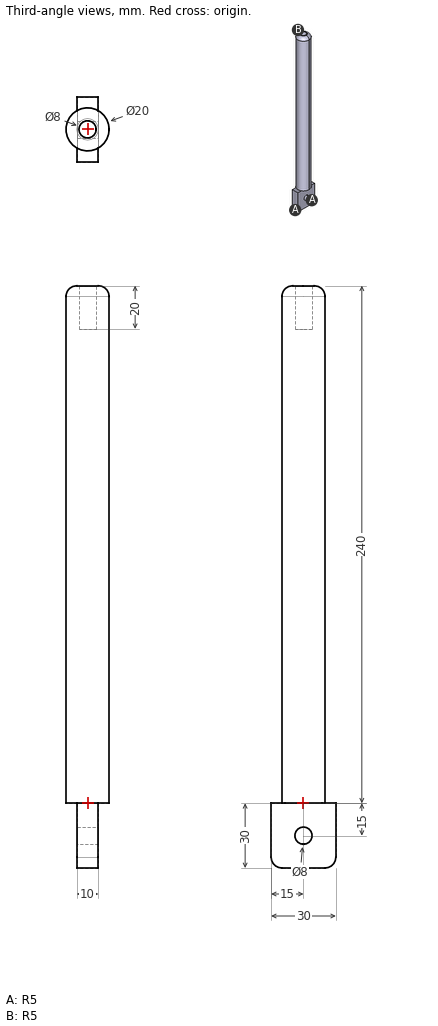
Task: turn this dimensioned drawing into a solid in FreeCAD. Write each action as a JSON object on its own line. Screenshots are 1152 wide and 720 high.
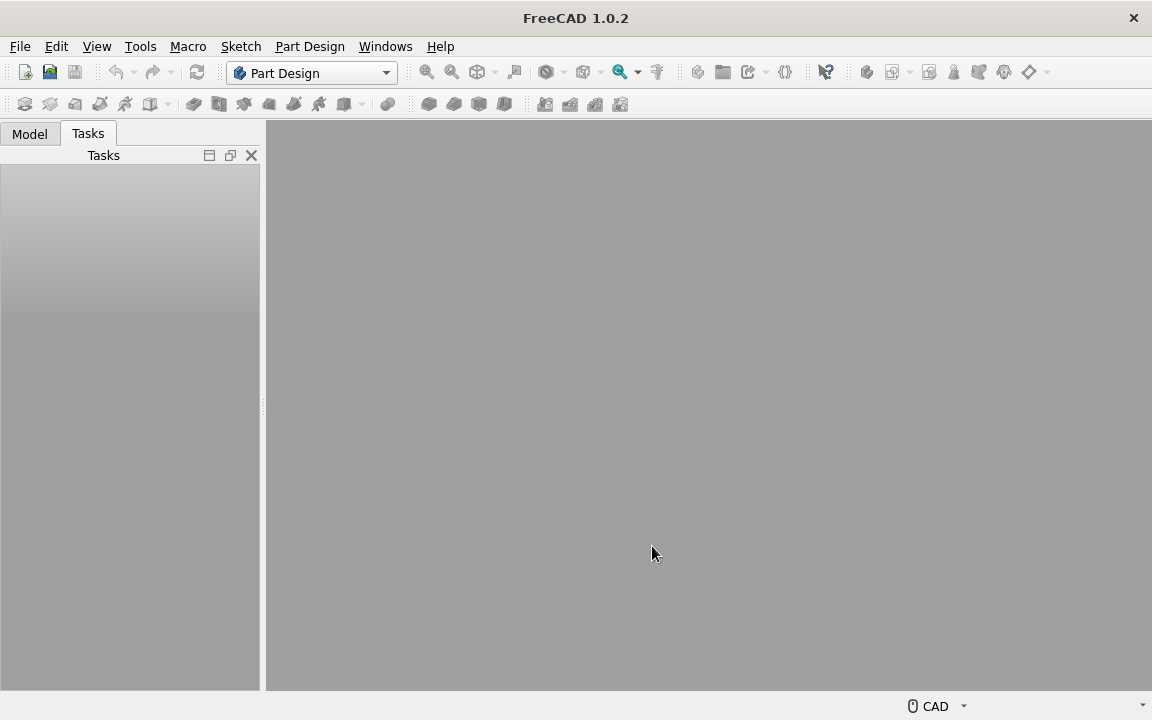
{"action": "key", "text": "ctrl+n"}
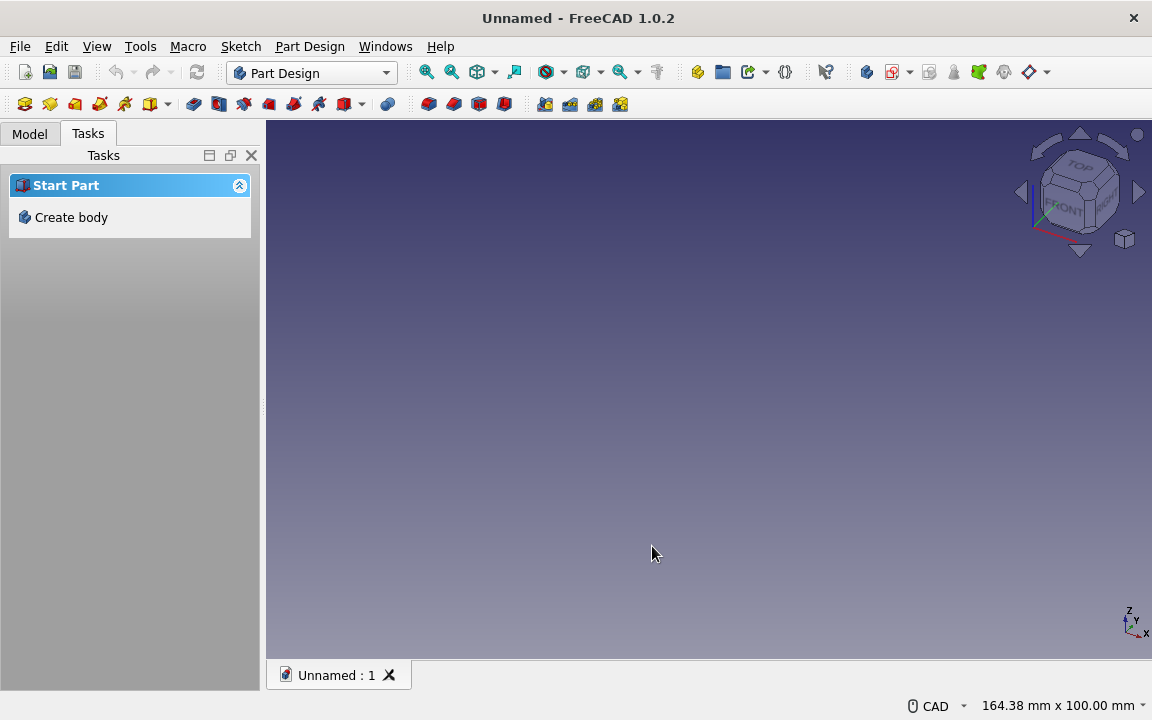
{"action": "left_click", "coordinate": [892, 72]}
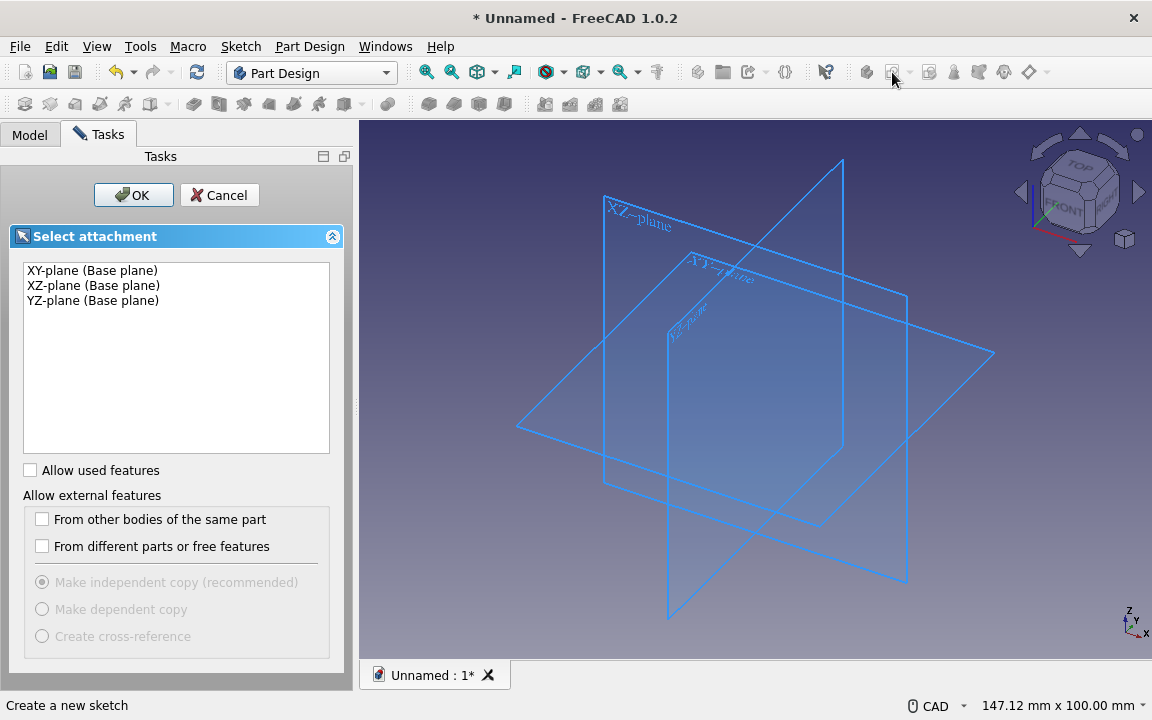
{"action": "left_click", "coordinate": [84, 270]}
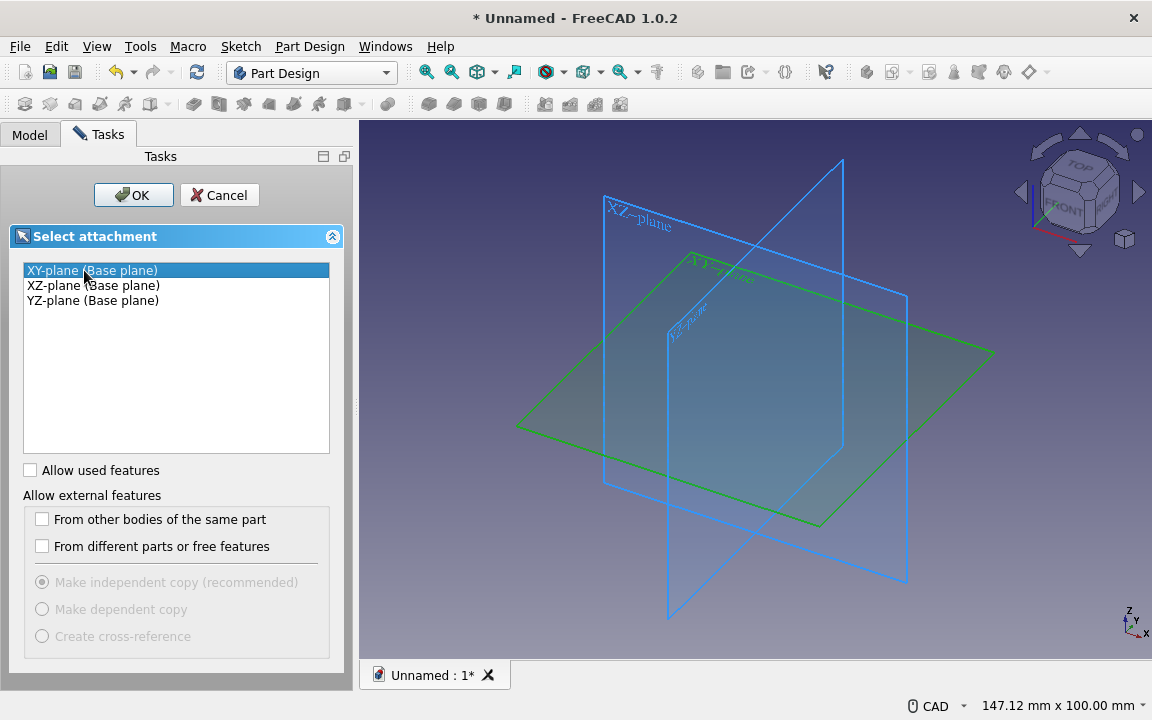
{"action": "left_click", "coordinate": [134, 195]}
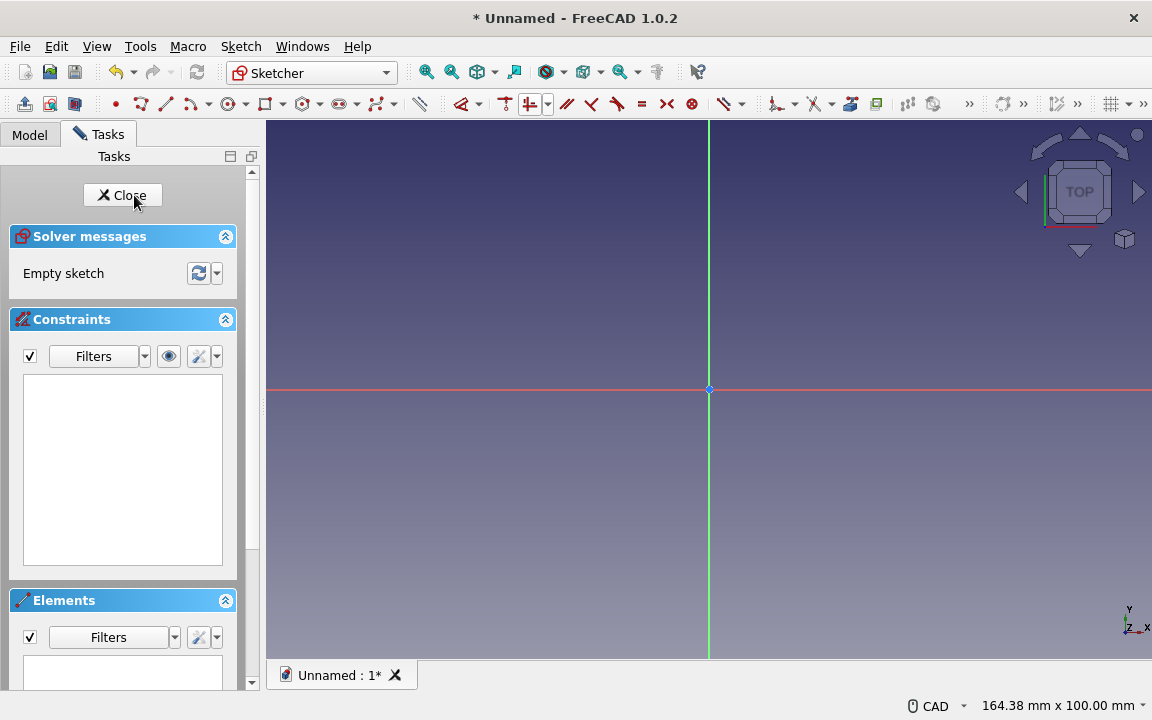
{"action": "scroll", "coordinate": [739, 390], "scroll_direction": "up", "scroll_amount": 6}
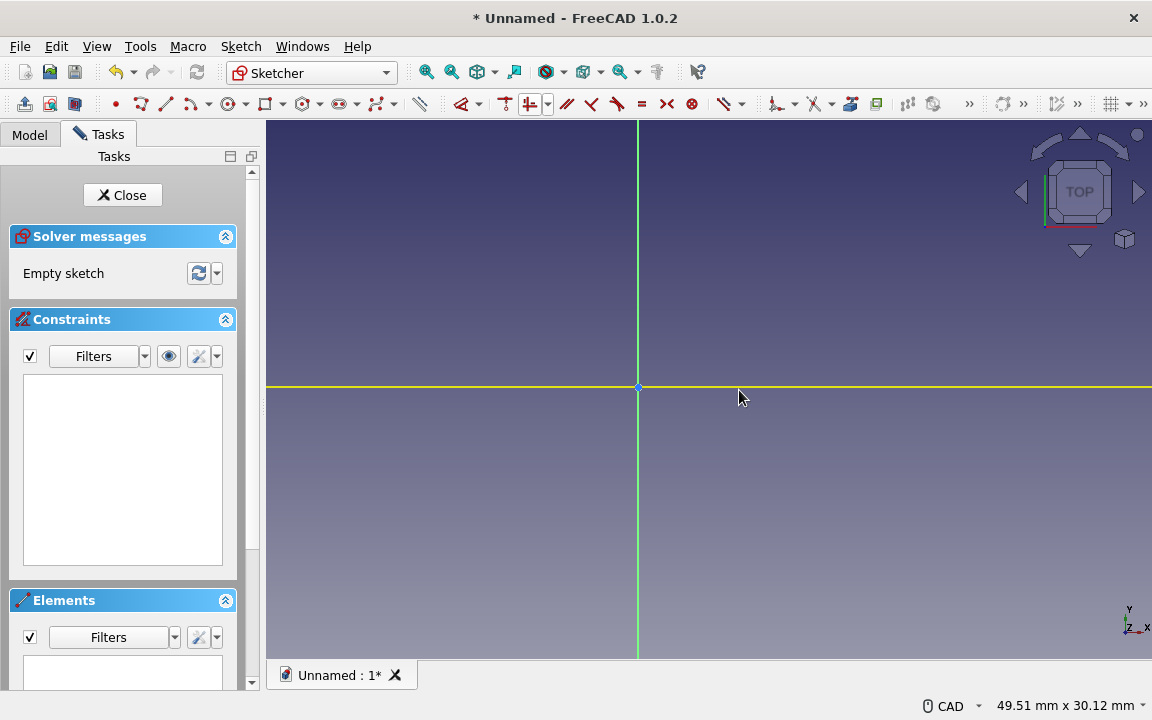
{"action": "left_click", "coordinate": [228, 104]}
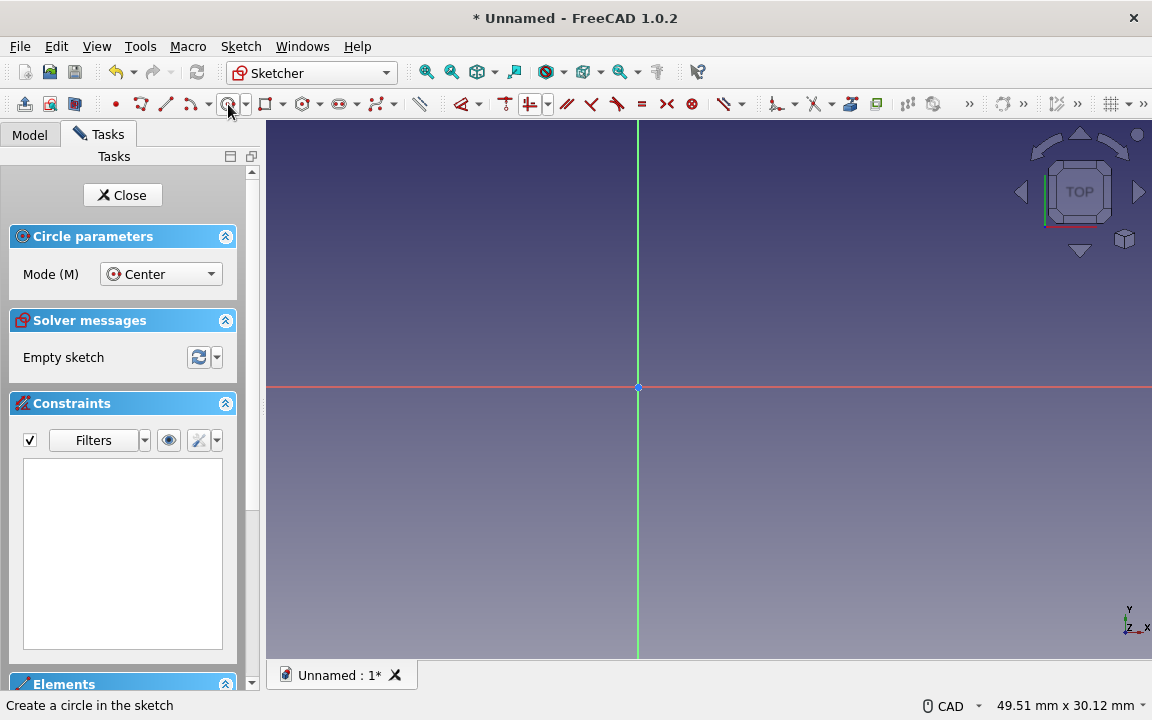
{"action": "left_click", "coordinate": [638, 387]}
{"action": "left_click", "coordinate": [765, 261]}
{"action": "key", "text": "Escape"}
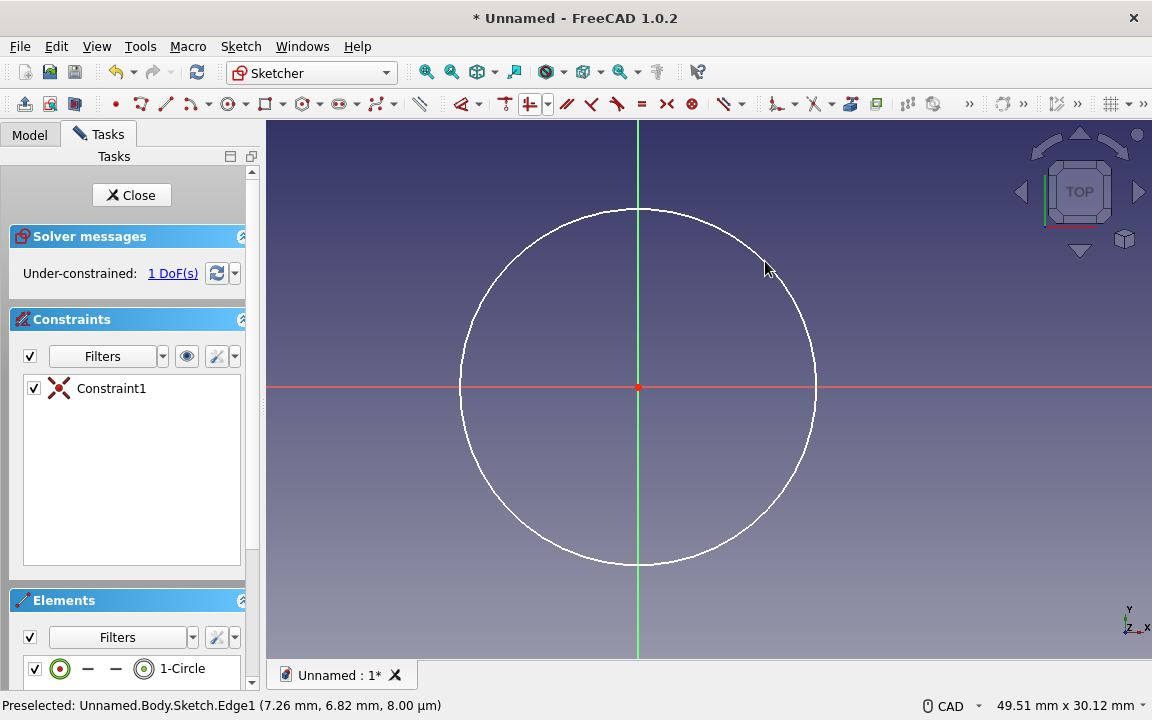
{"action": "left_click", "coordinate": [460, 104]}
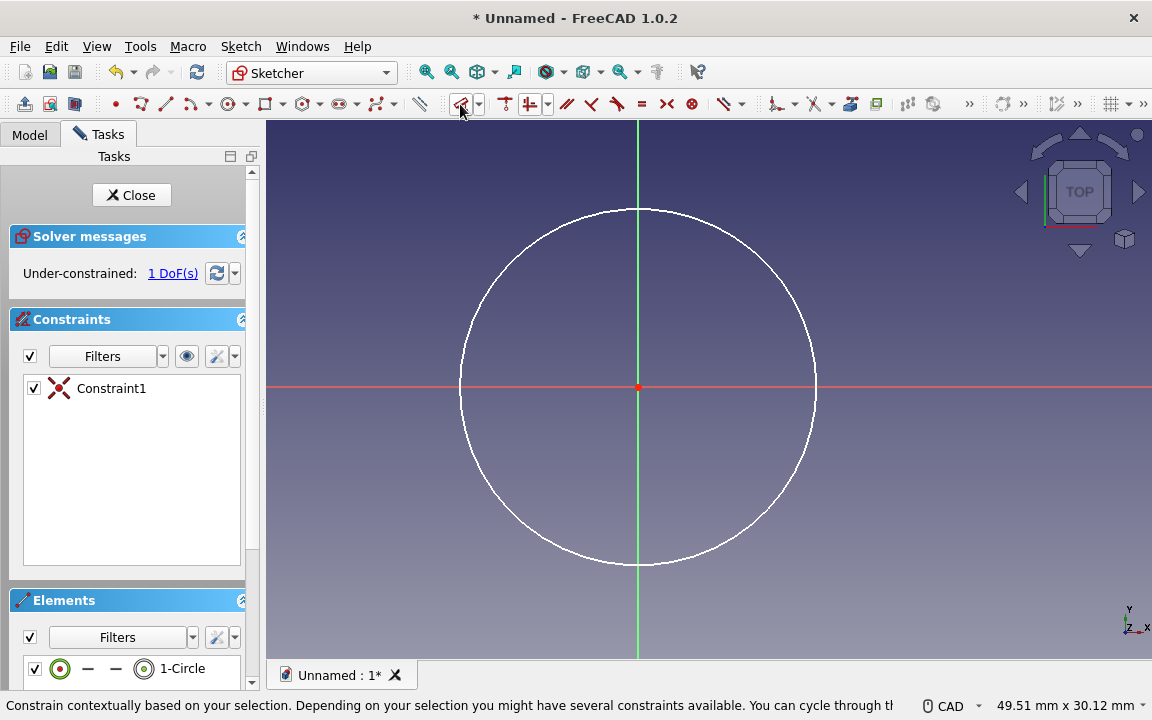
{"action": "left_click", "coordinate": [764, 261]}
{"action": "left_click", "coordinate": [787, 238]}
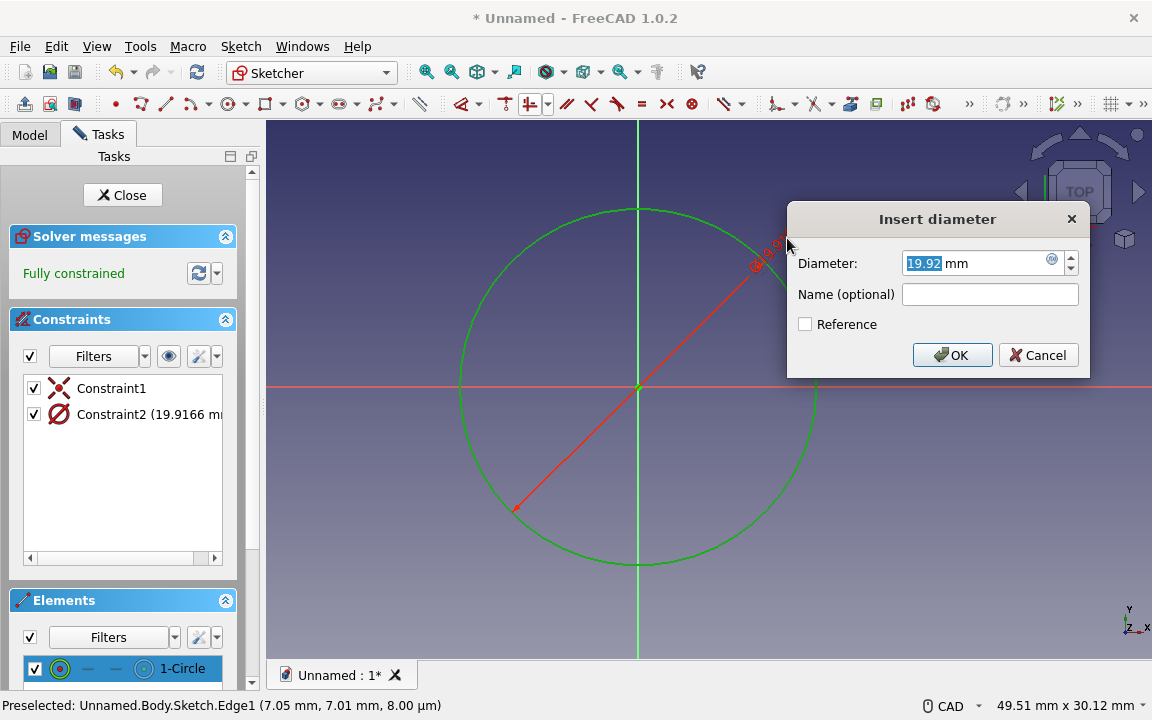
{"action": "type", "text": "20"}
{"action": "key", "text": "Return"}
{"action": "key", "text": "Escape"}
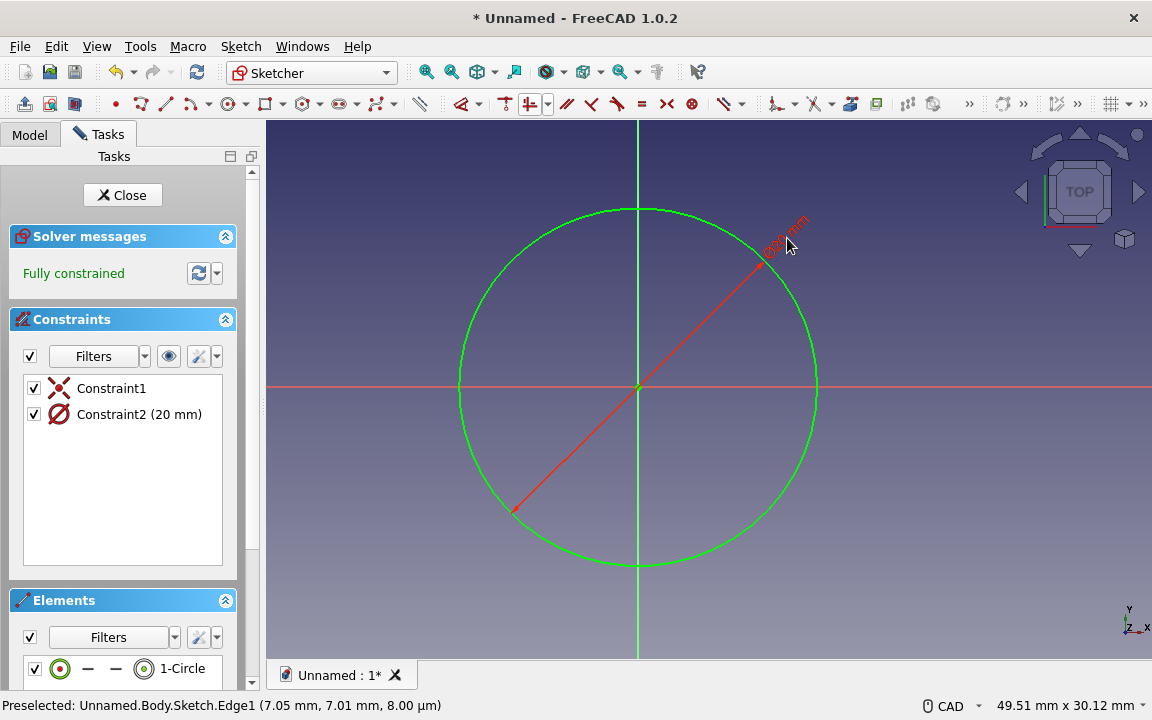
{"action": "left_click", "coordinate": [123, 195]}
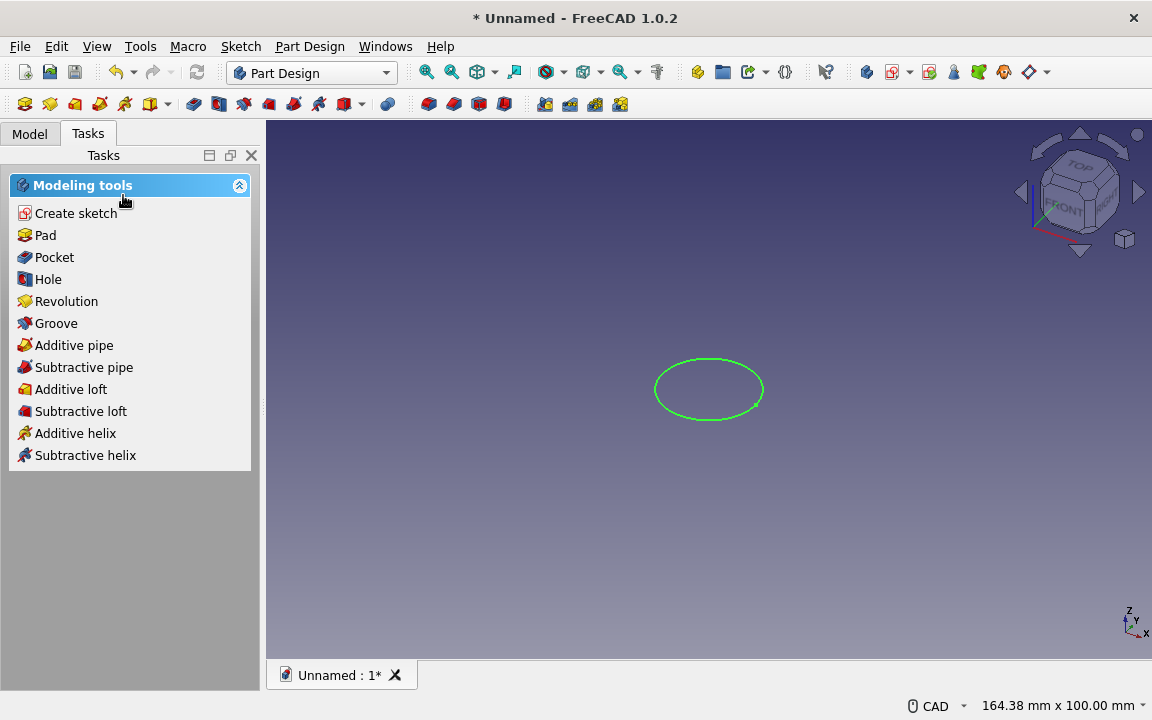
{"action": "left_click", "coordinate": [25, 104]}